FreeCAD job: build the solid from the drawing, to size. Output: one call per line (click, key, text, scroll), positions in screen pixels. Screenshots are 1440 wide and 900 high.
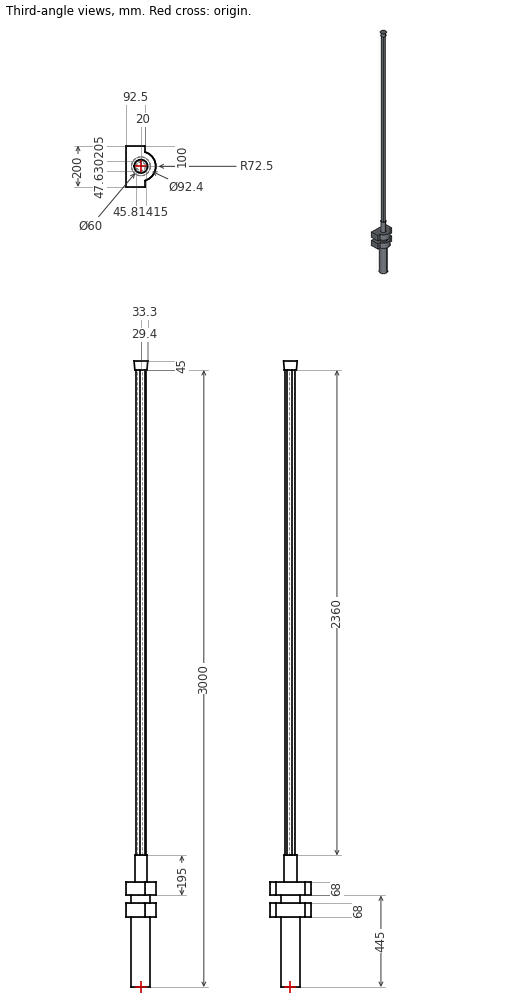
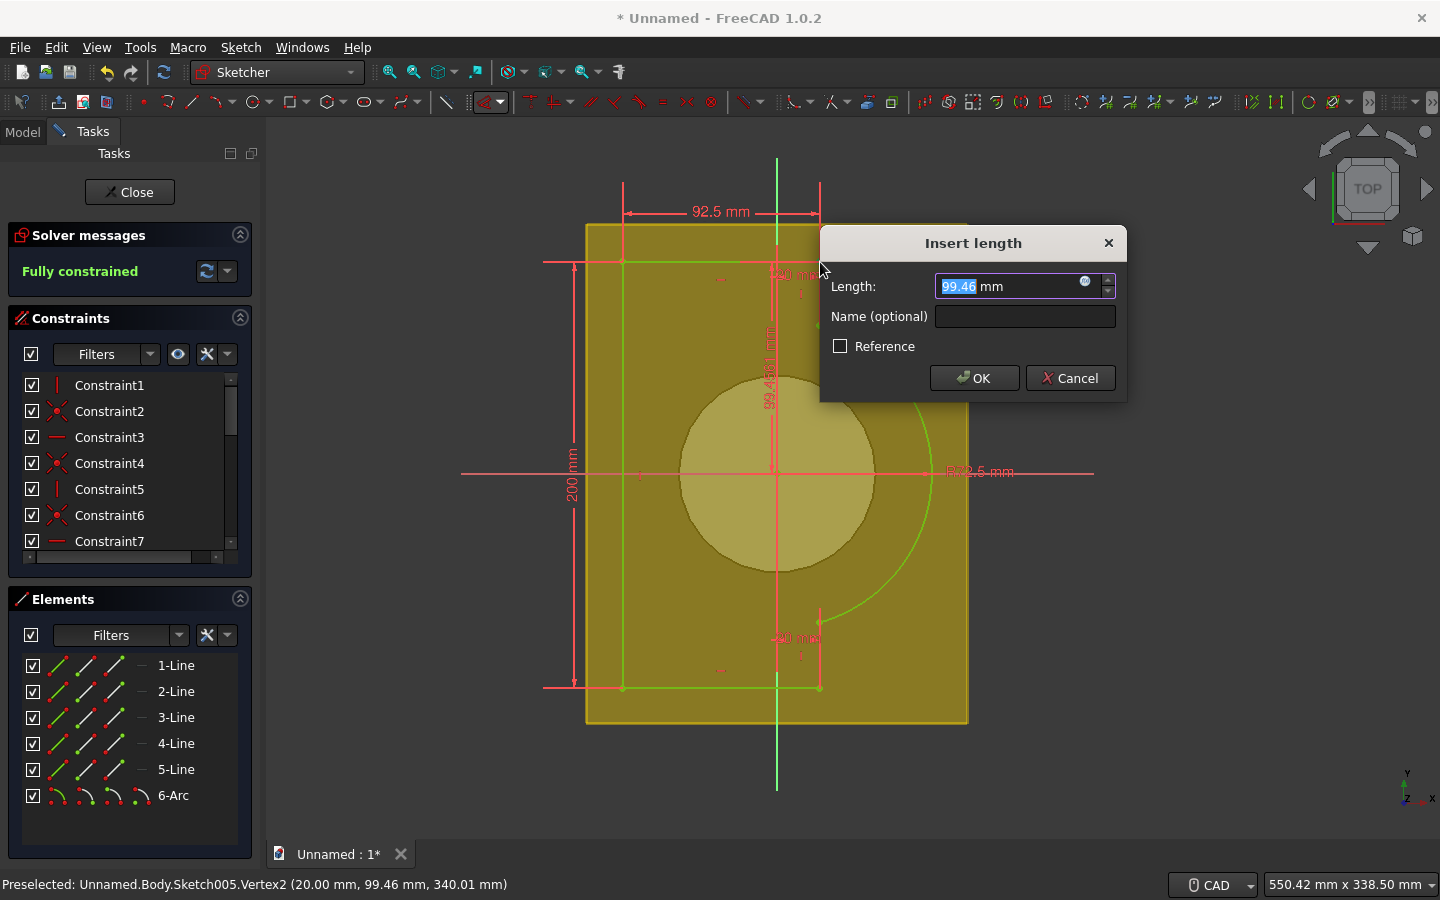
text(100)
key(Return)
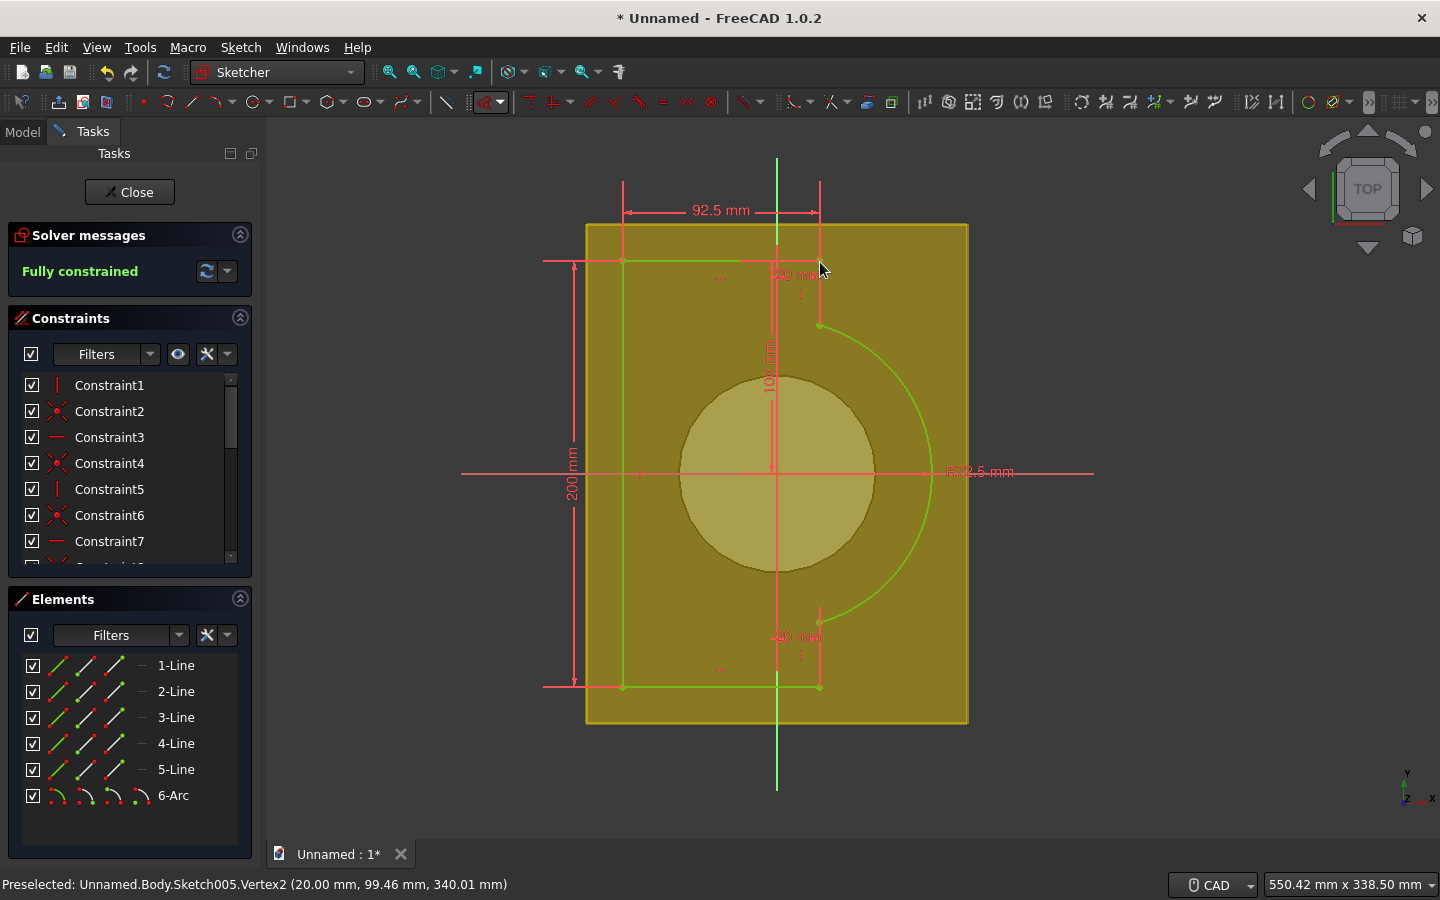
click(130, 192)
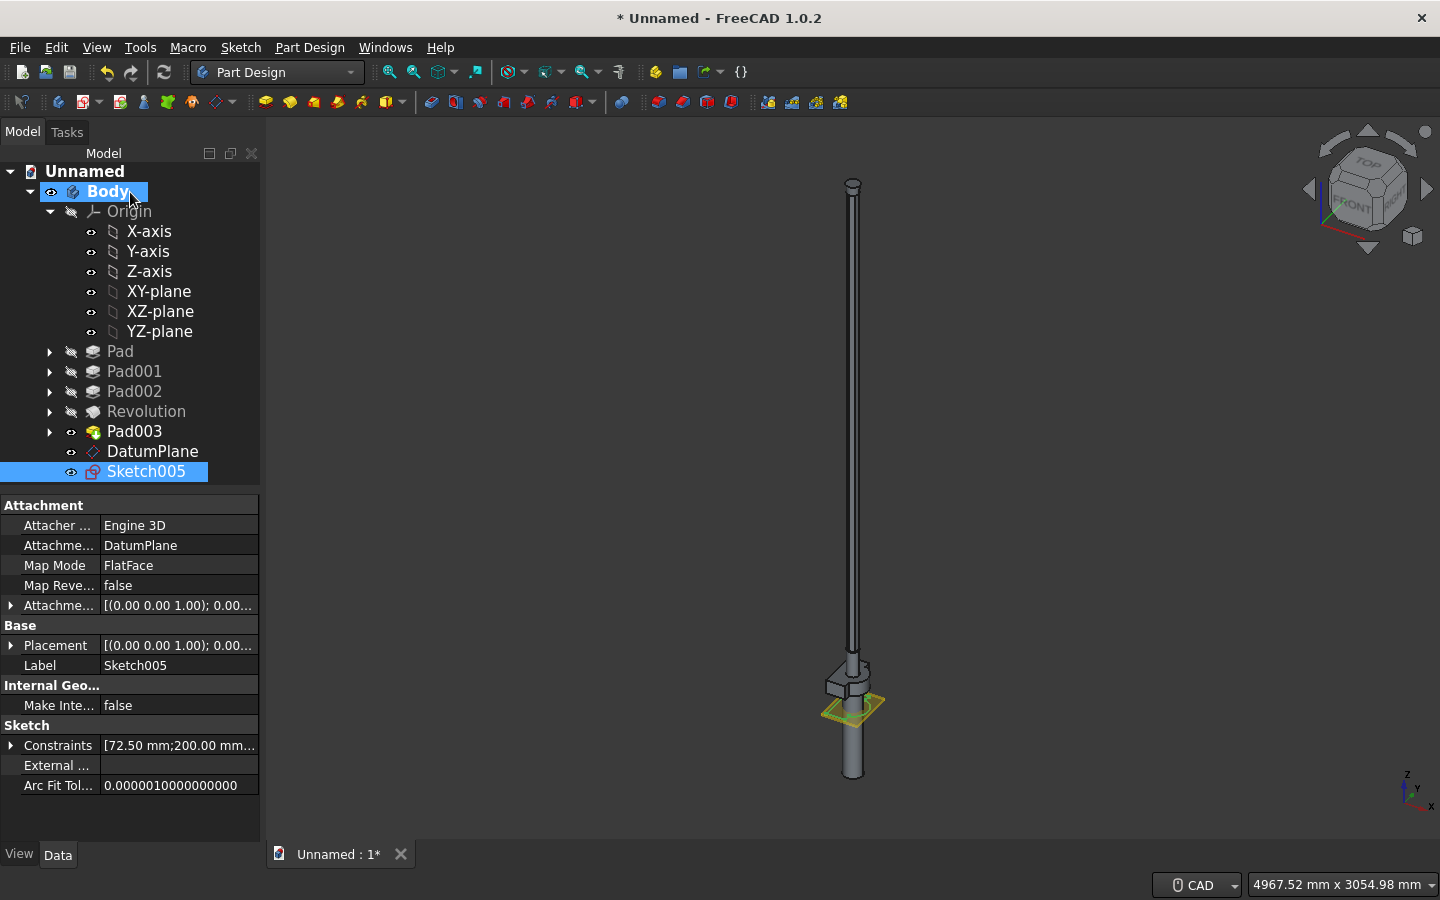
click(266, 102)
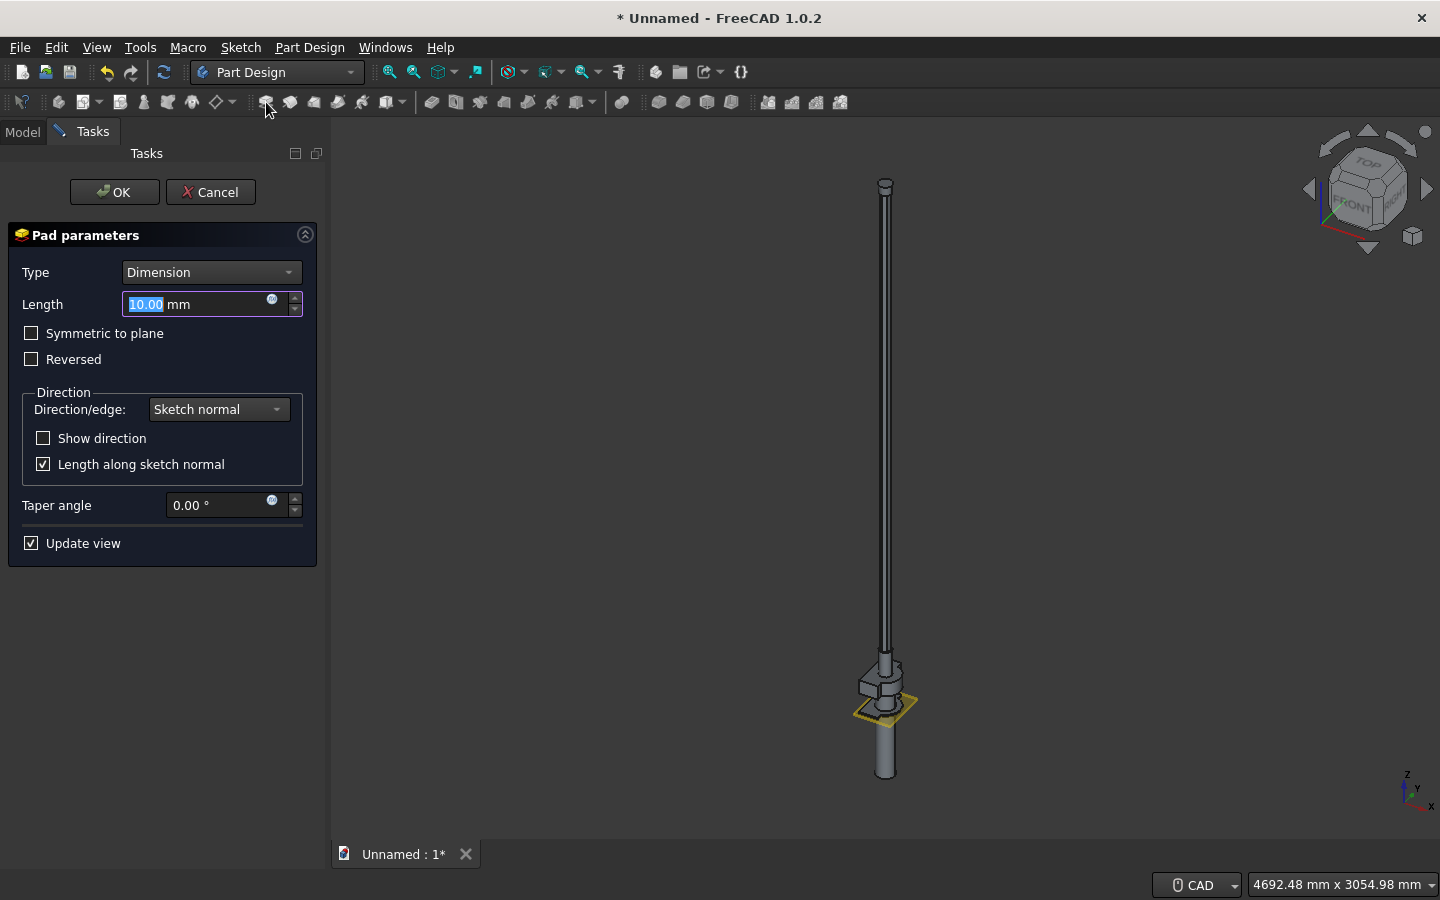
text(68)
key(Tab)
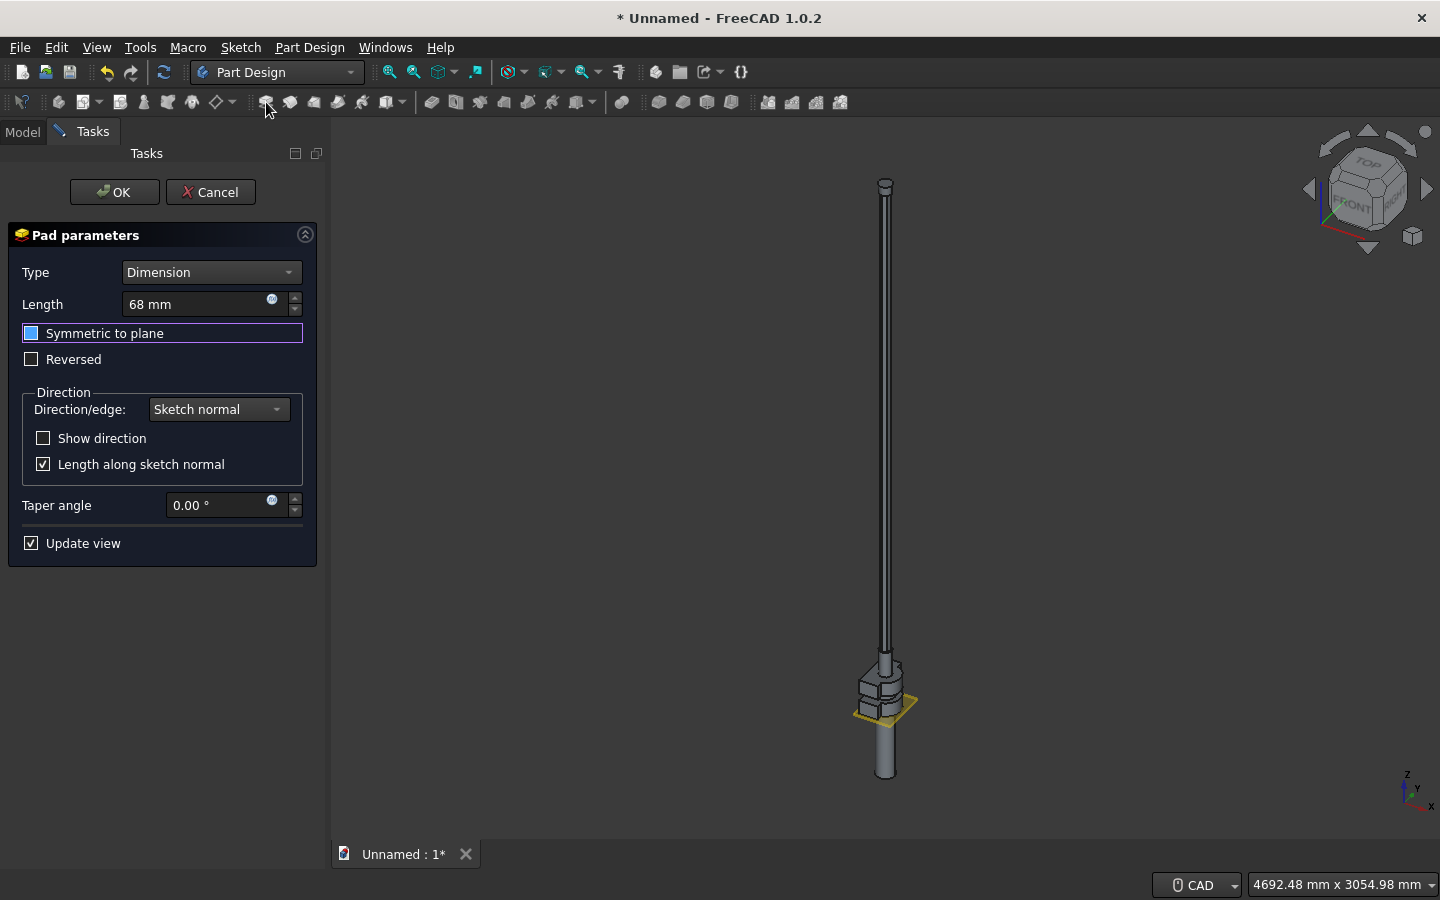
click(115, 192)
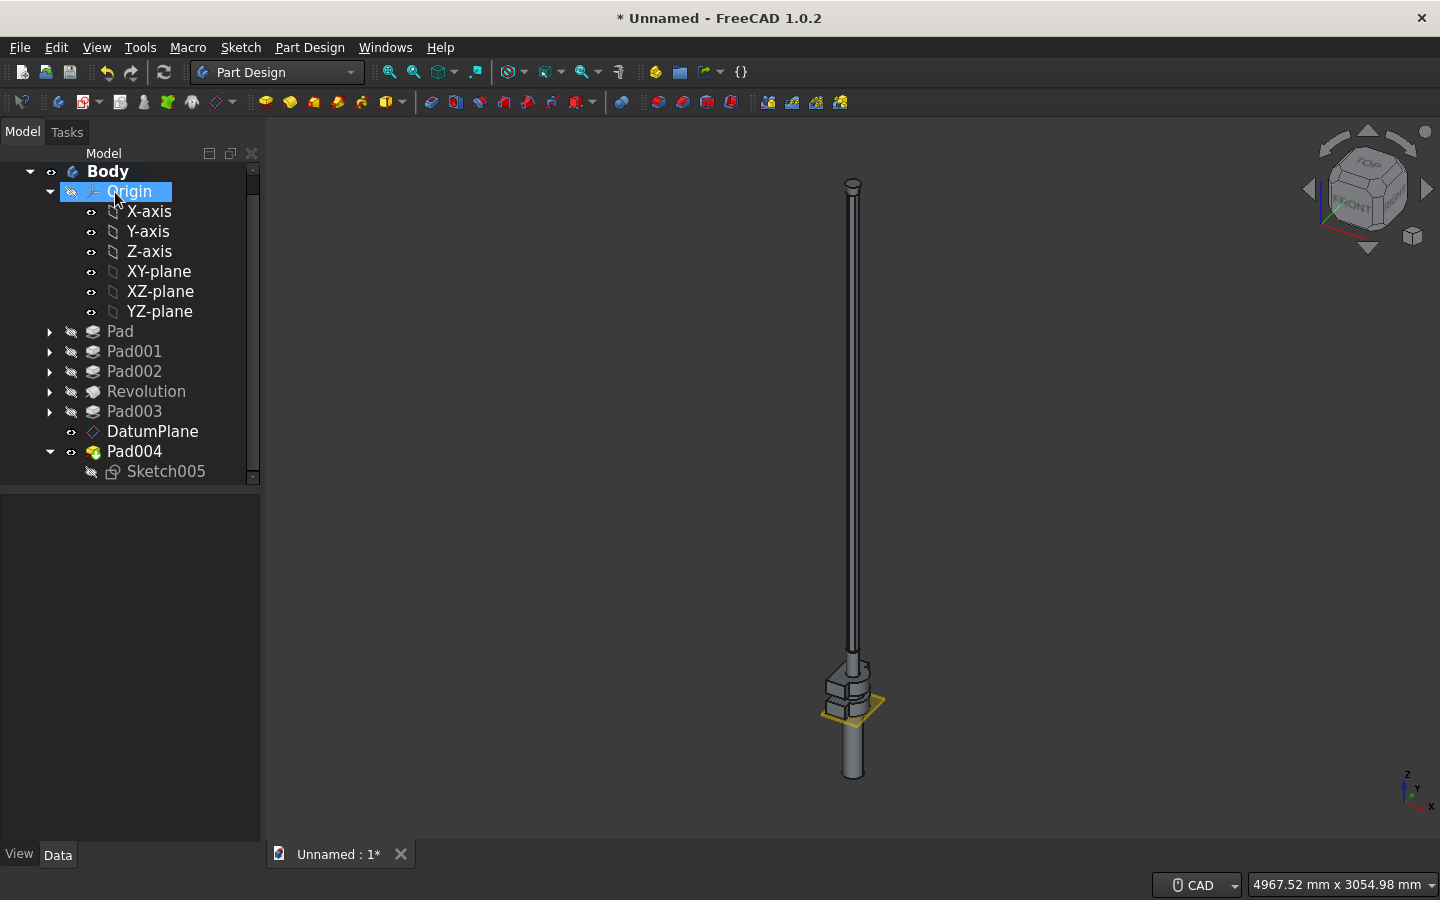
click(116, 432)
key(space)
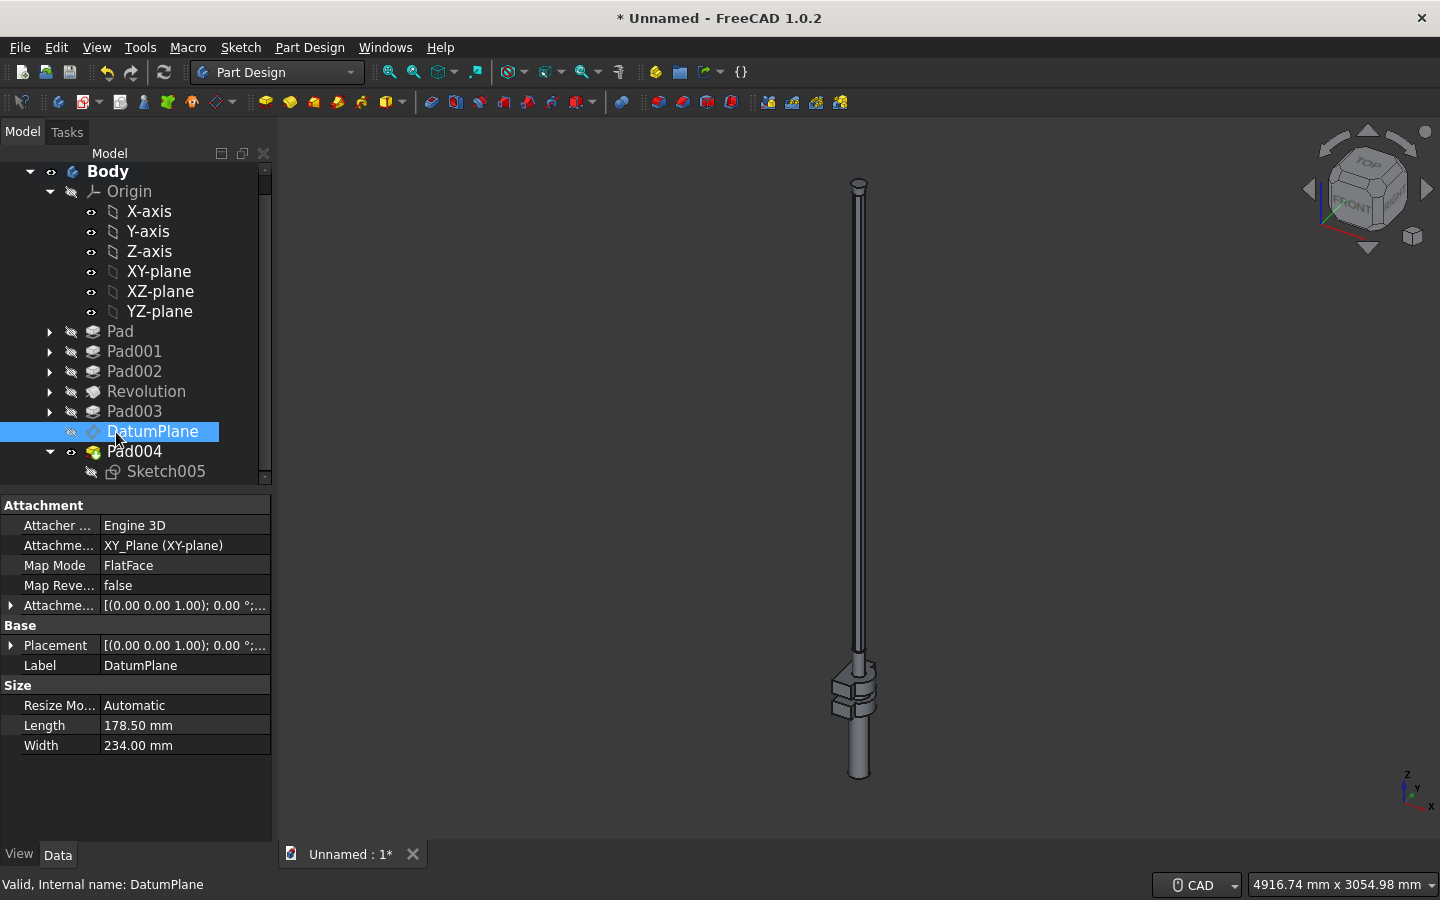
key(0)